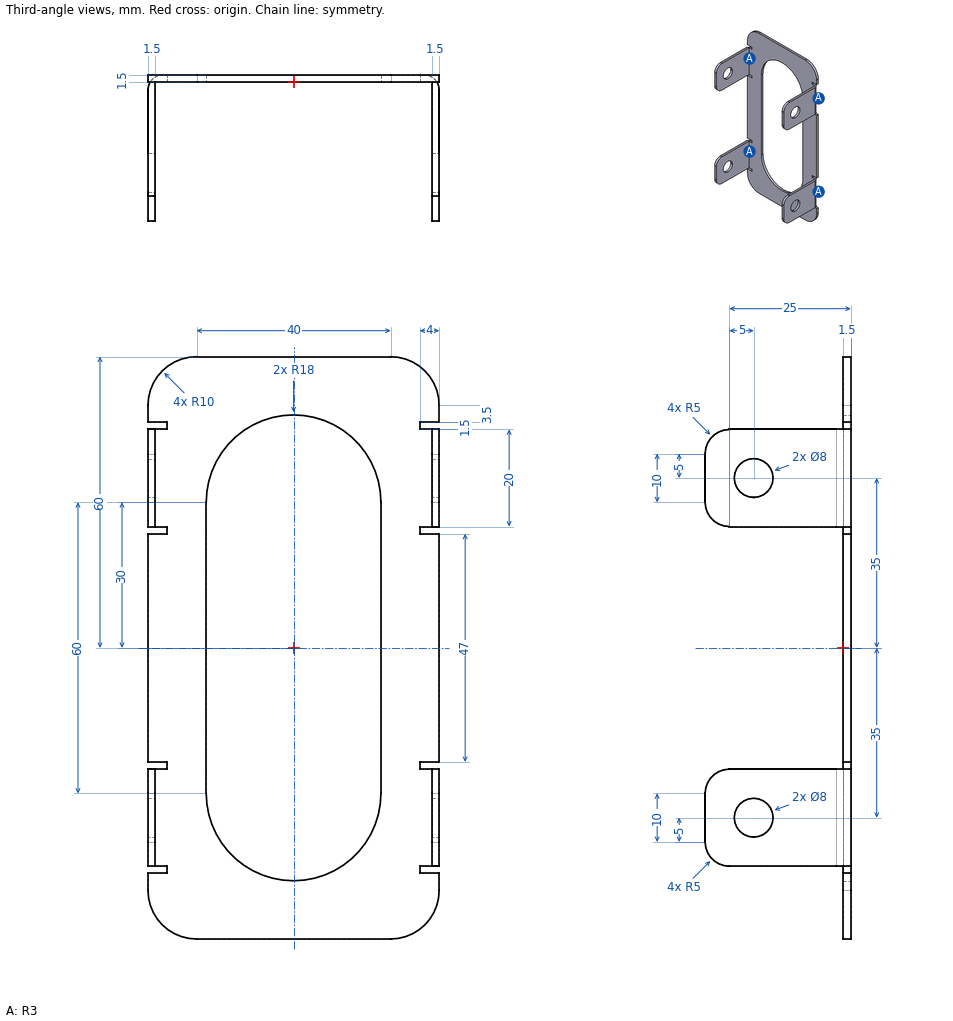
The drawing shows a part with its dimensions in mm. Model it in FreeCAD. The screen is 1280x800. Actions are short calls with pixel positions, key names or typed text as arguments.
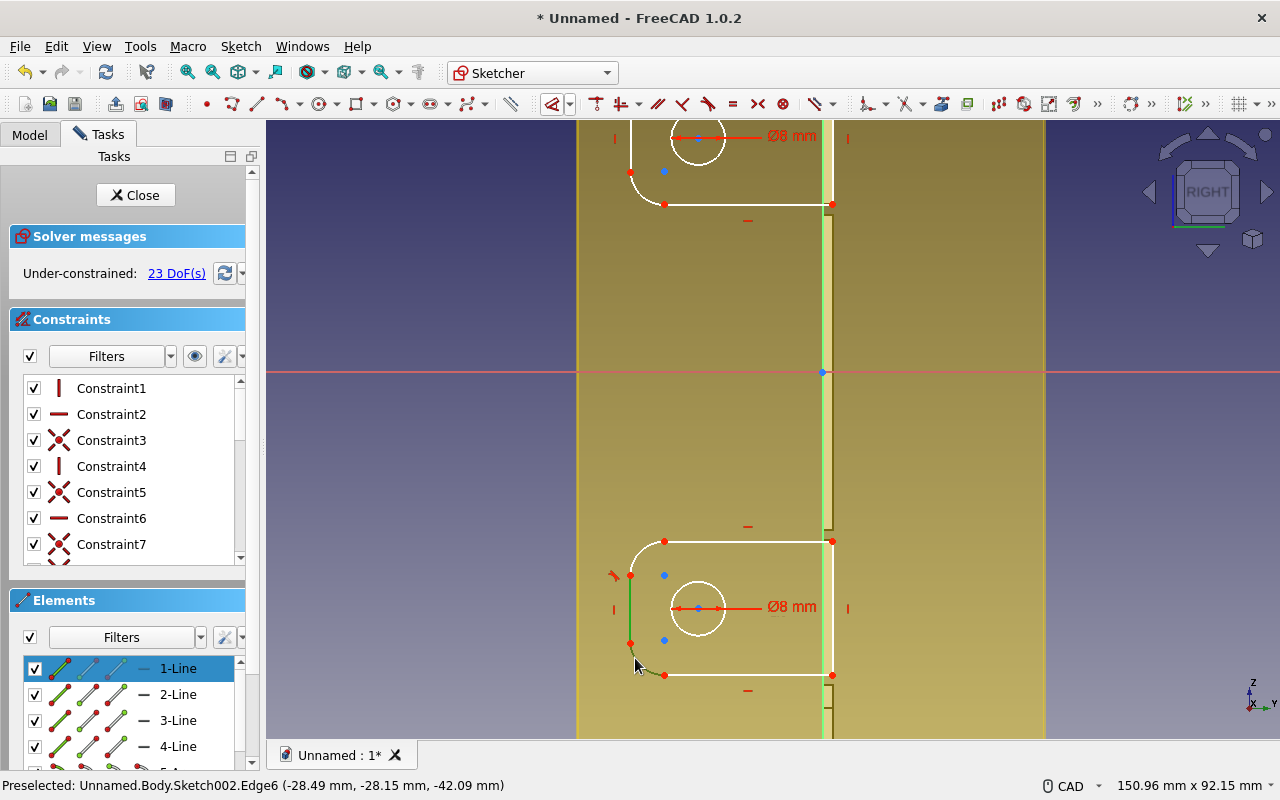
click(708, 104)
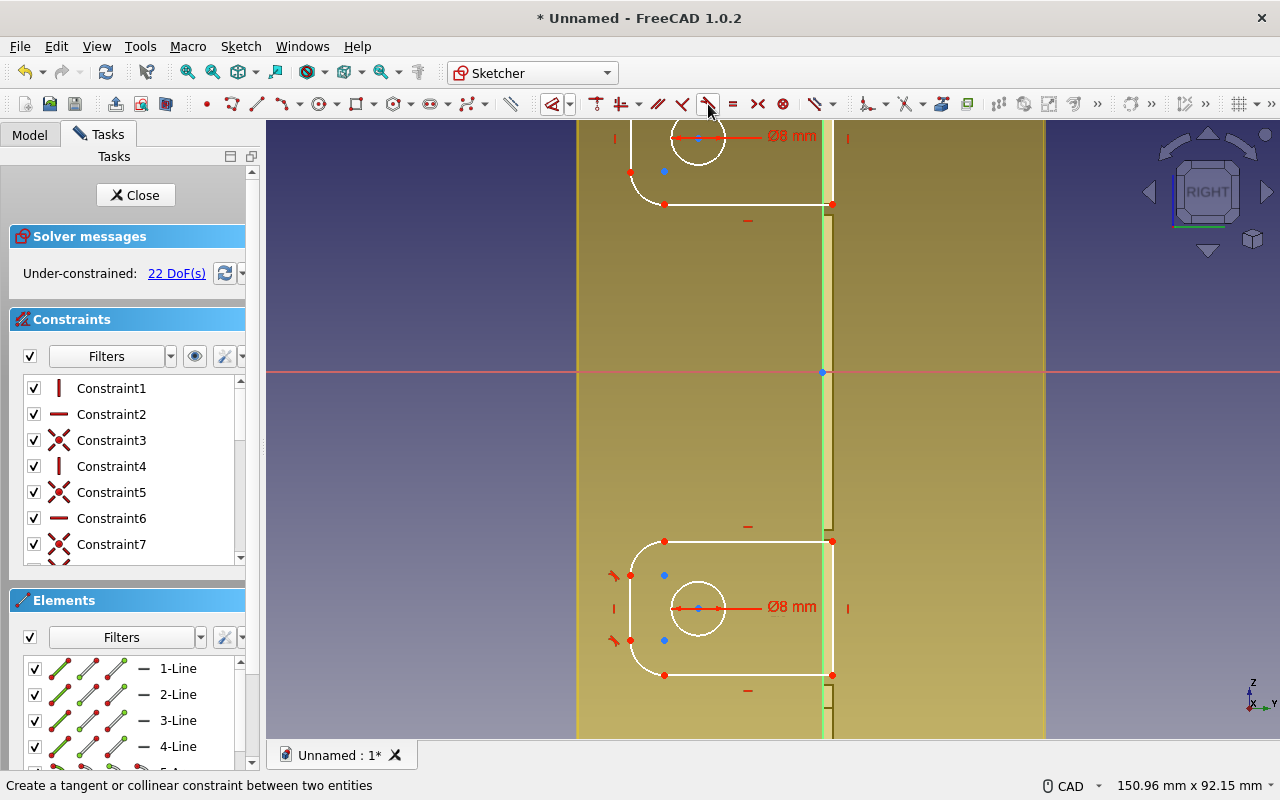
click(715, 542)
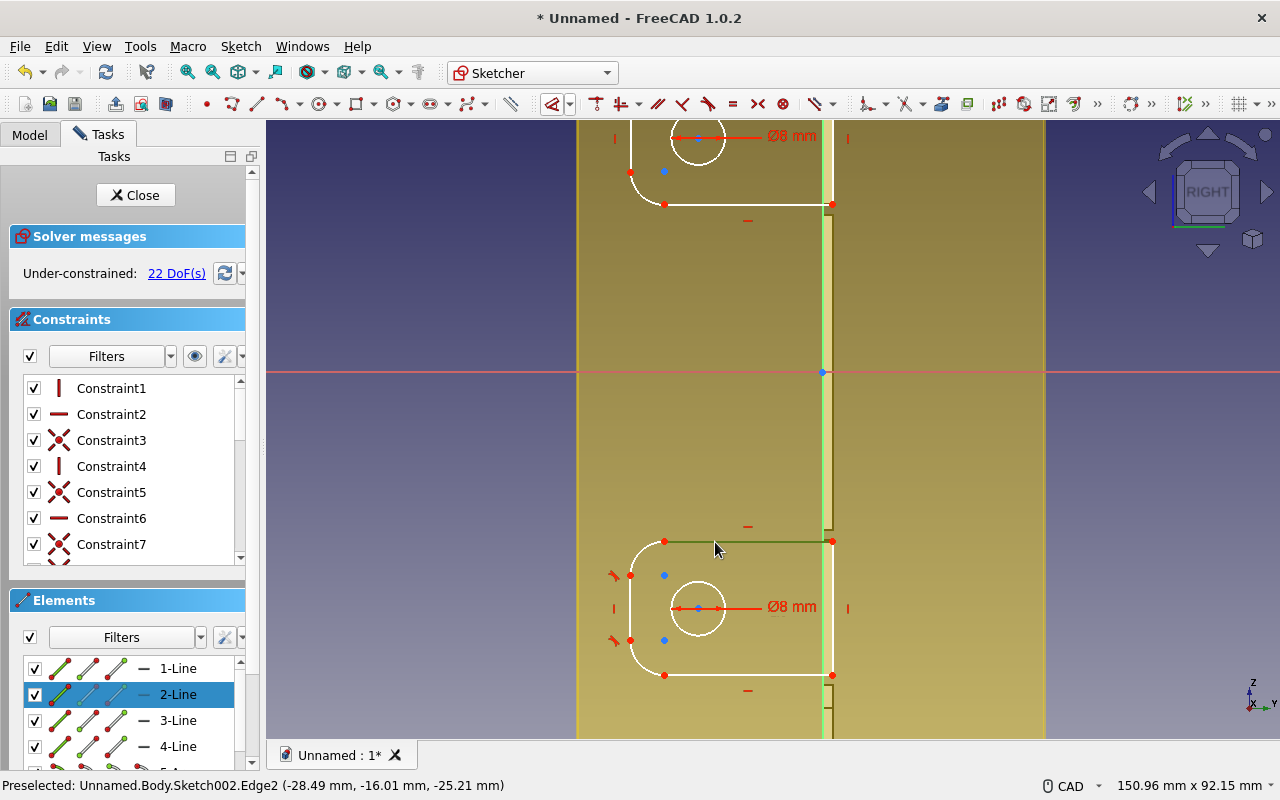
click(649, 545)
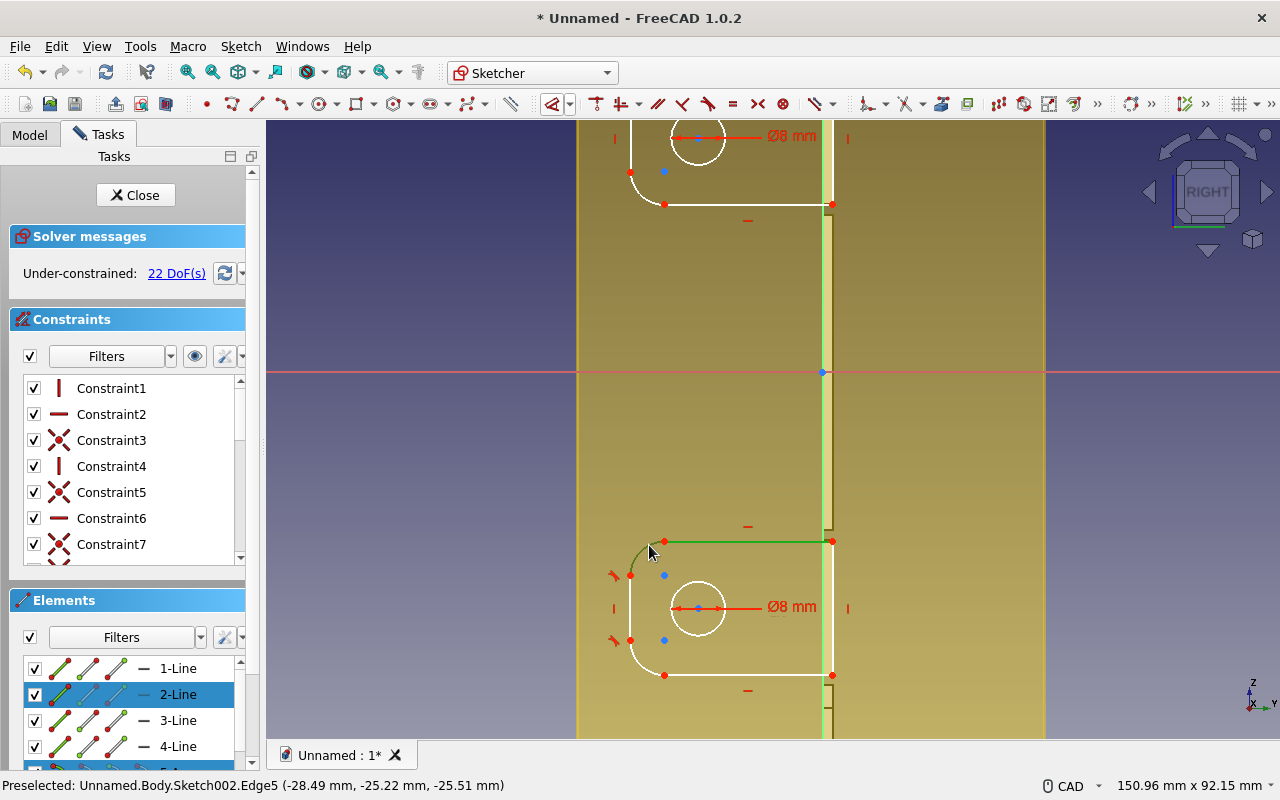
click(708, 104)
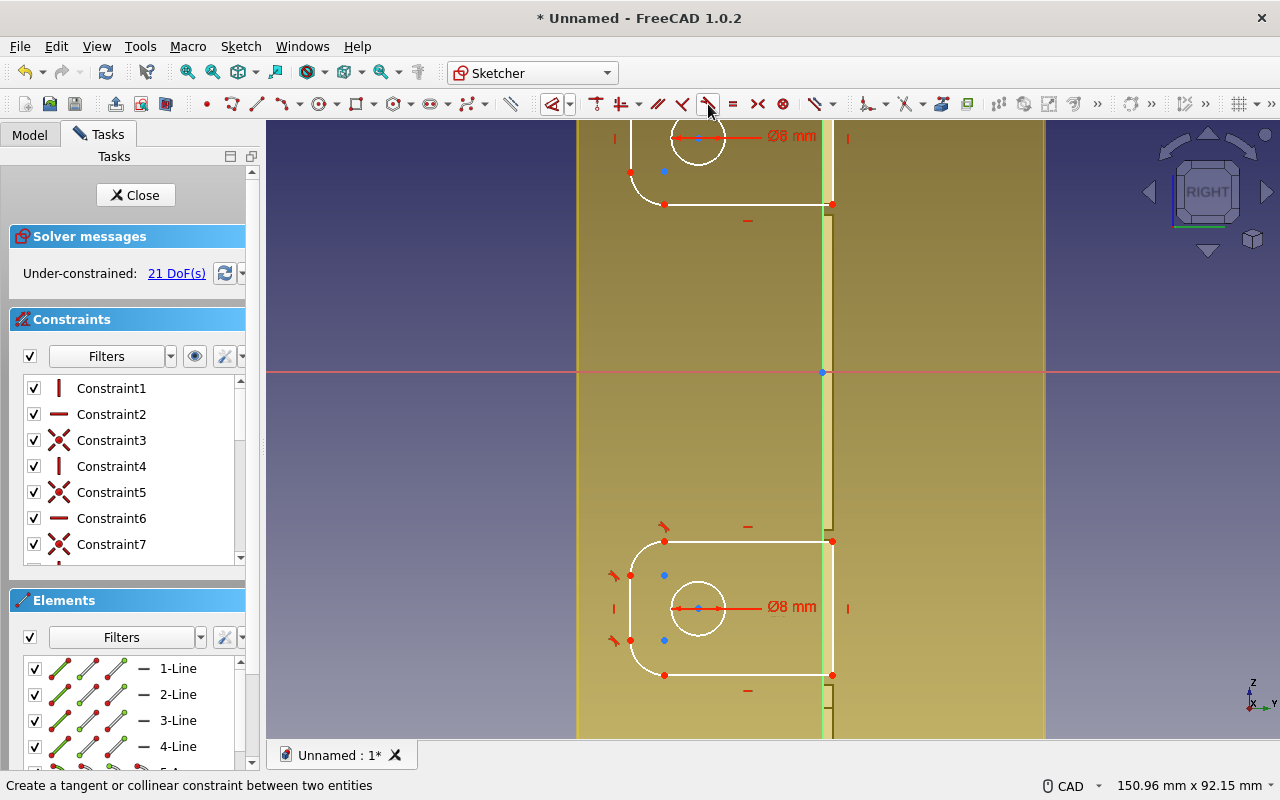
click(782, 675)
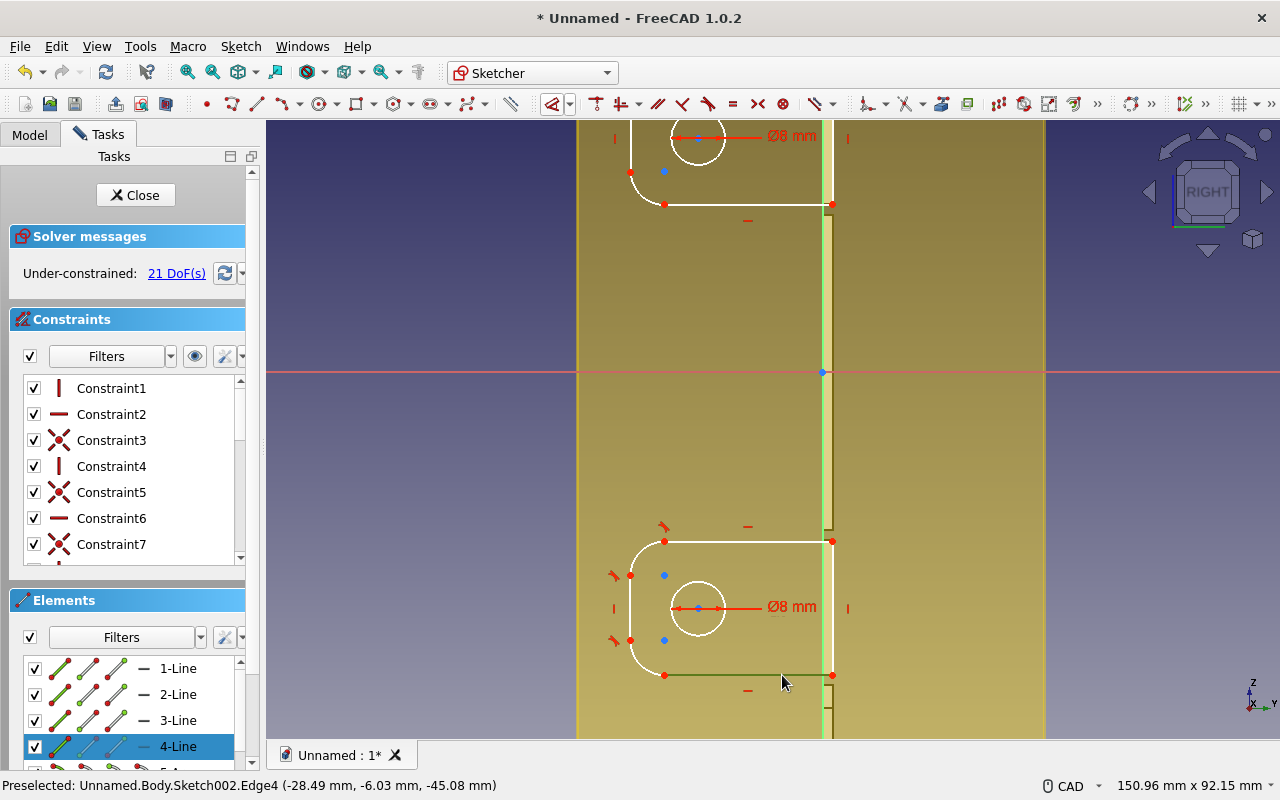
click(634, 656)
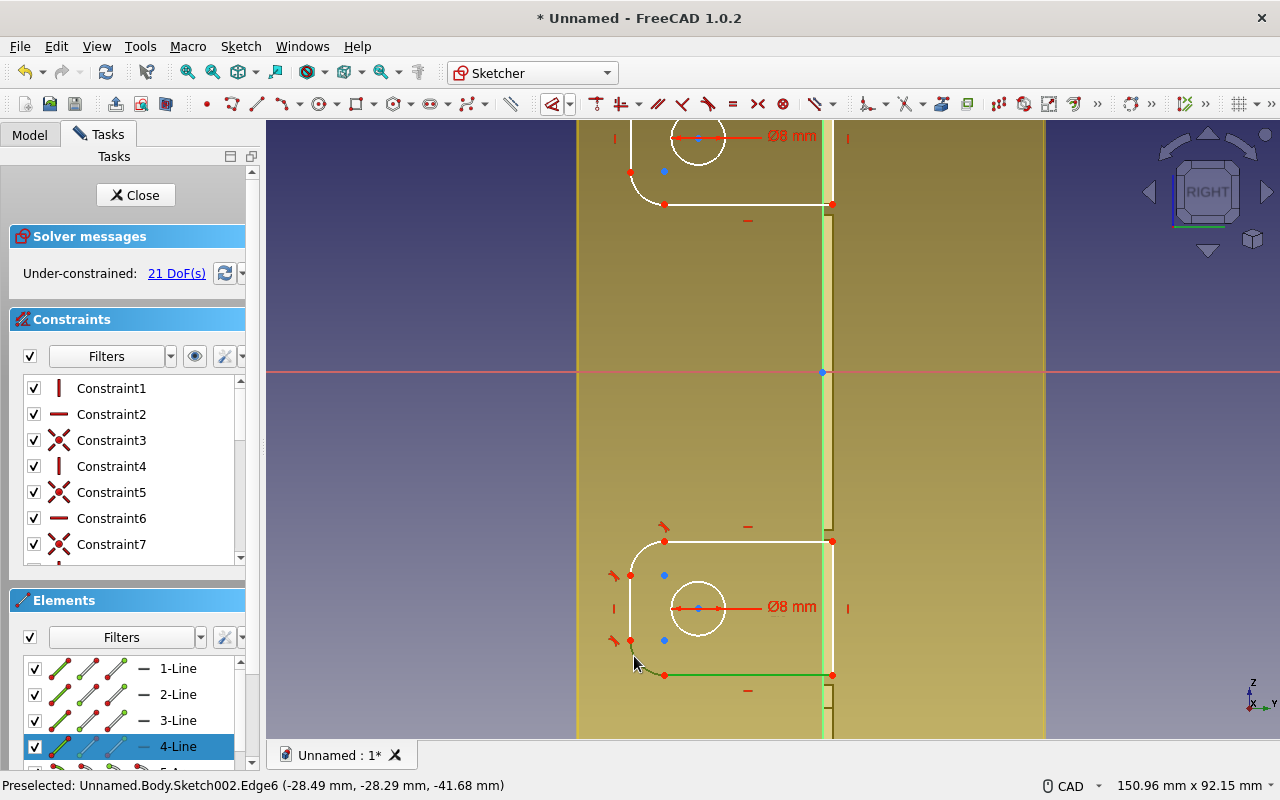
click(708, 104)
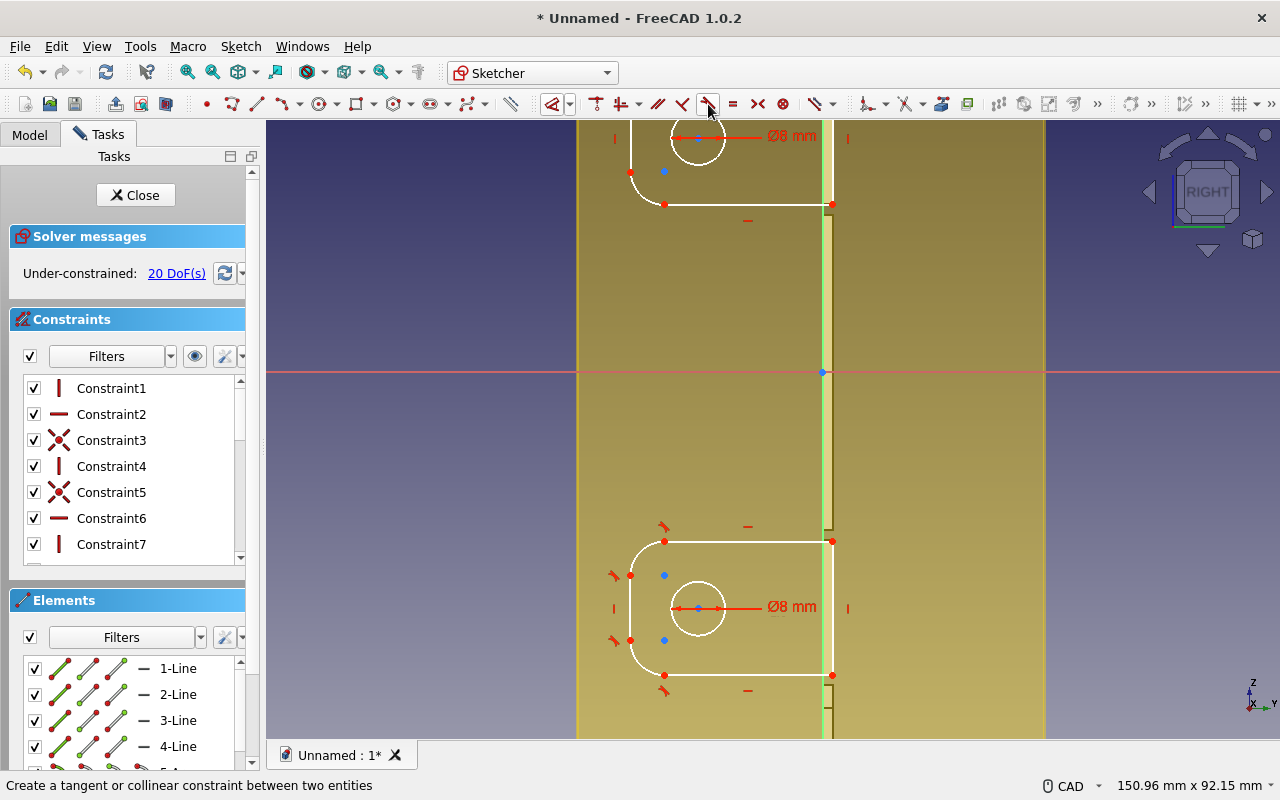
click(631, 152)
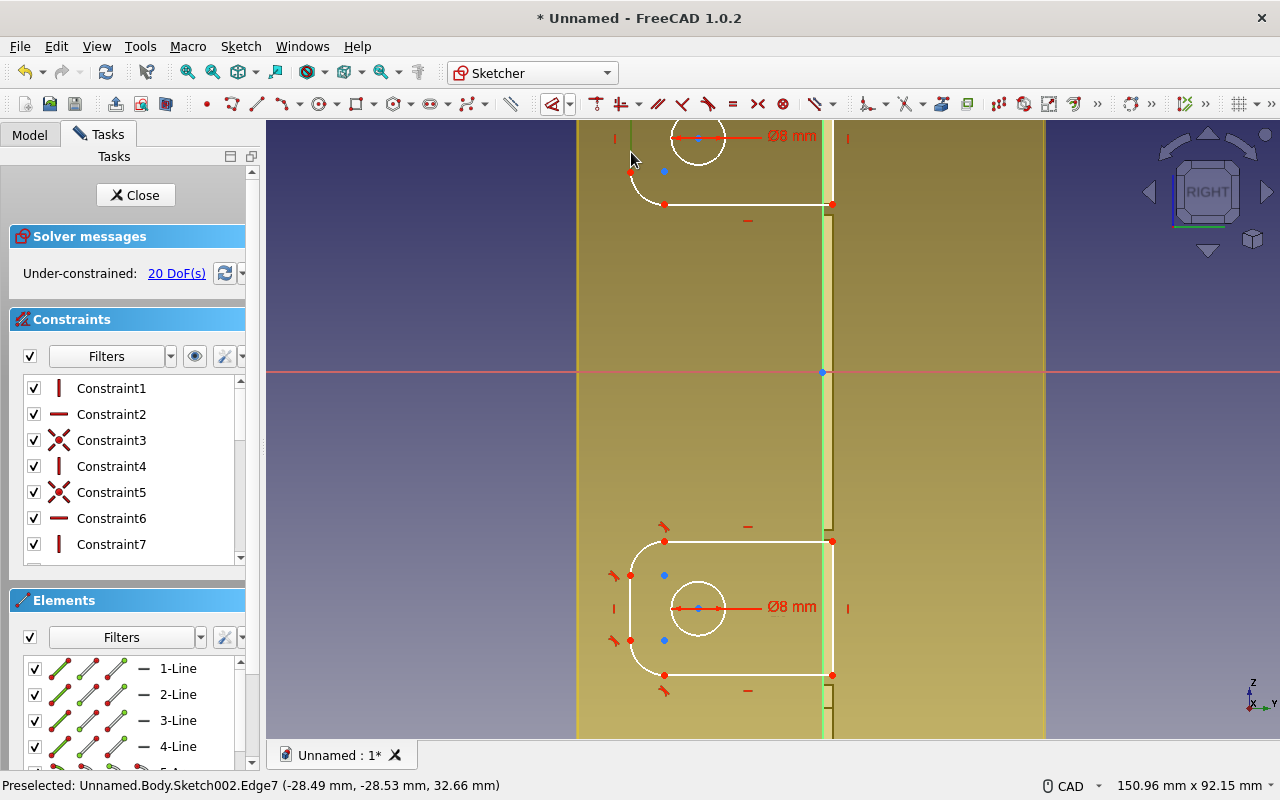
scroll(649, 546, down, 2)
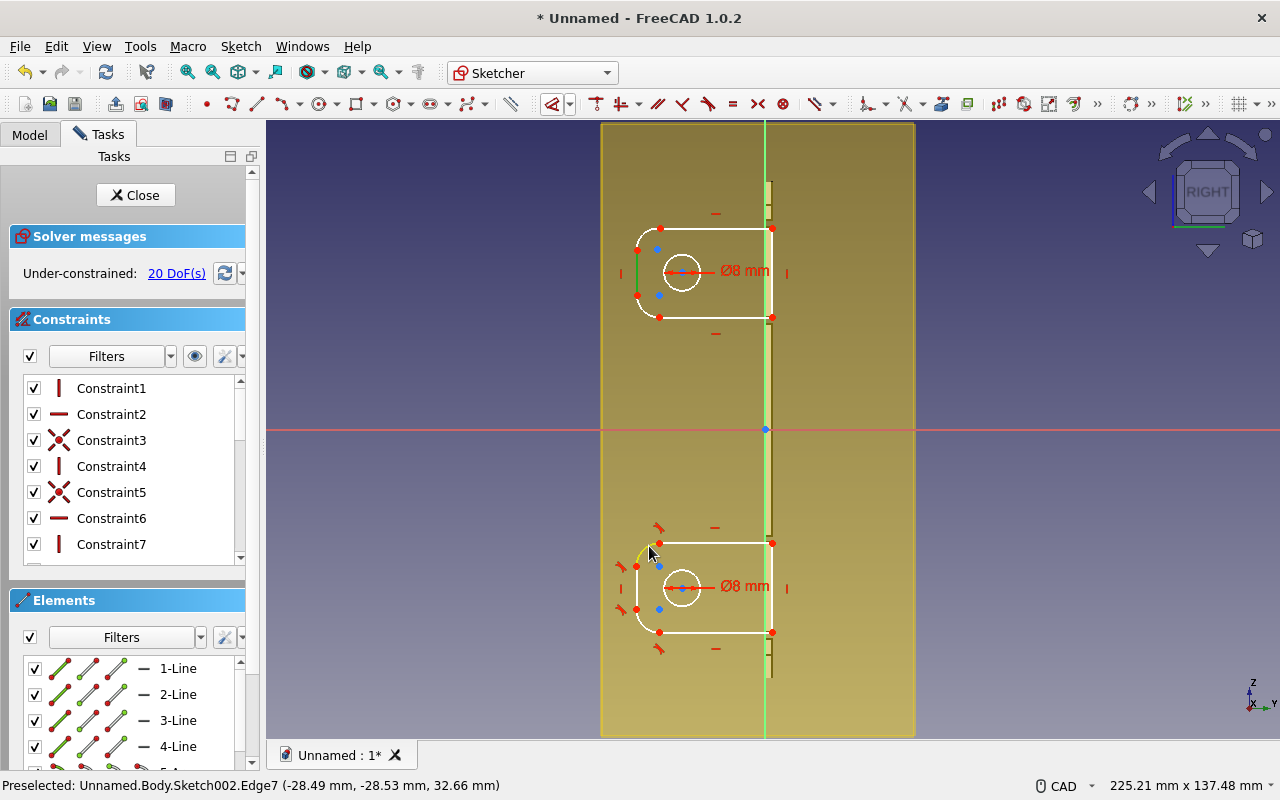
scroll(649, 230, up, 2)